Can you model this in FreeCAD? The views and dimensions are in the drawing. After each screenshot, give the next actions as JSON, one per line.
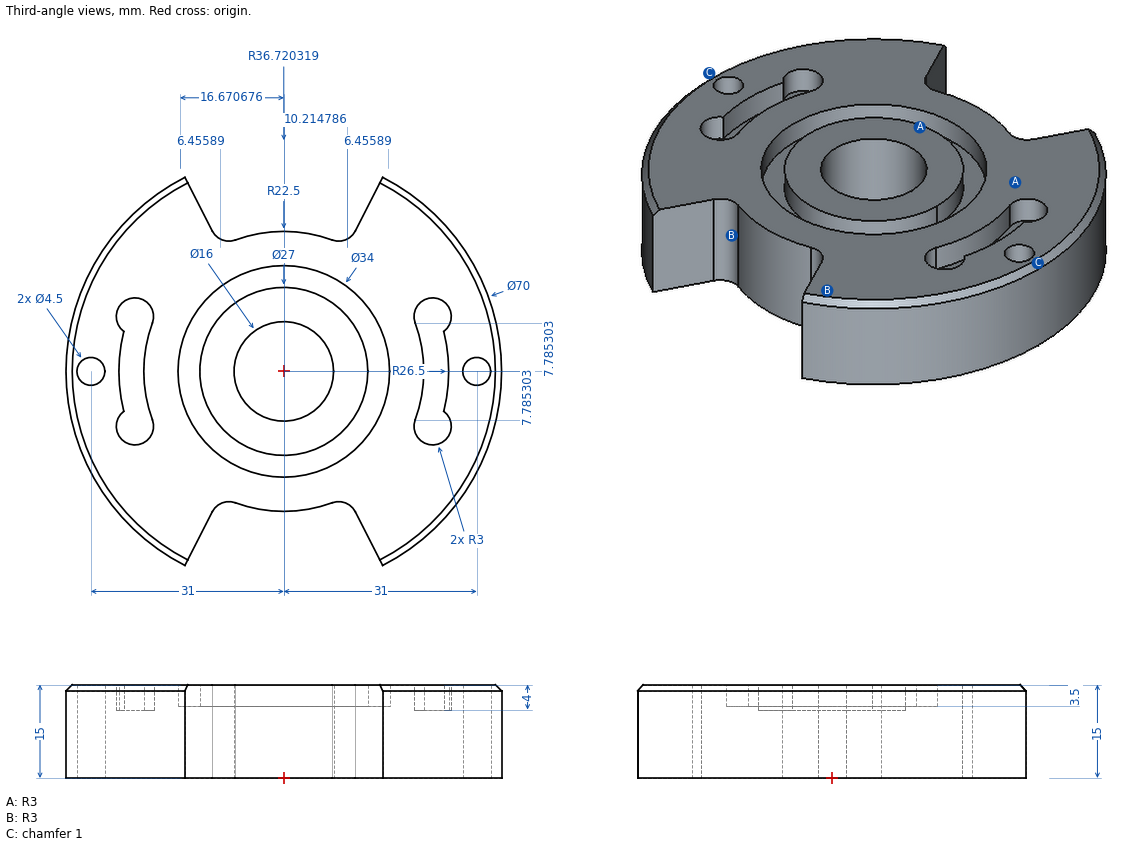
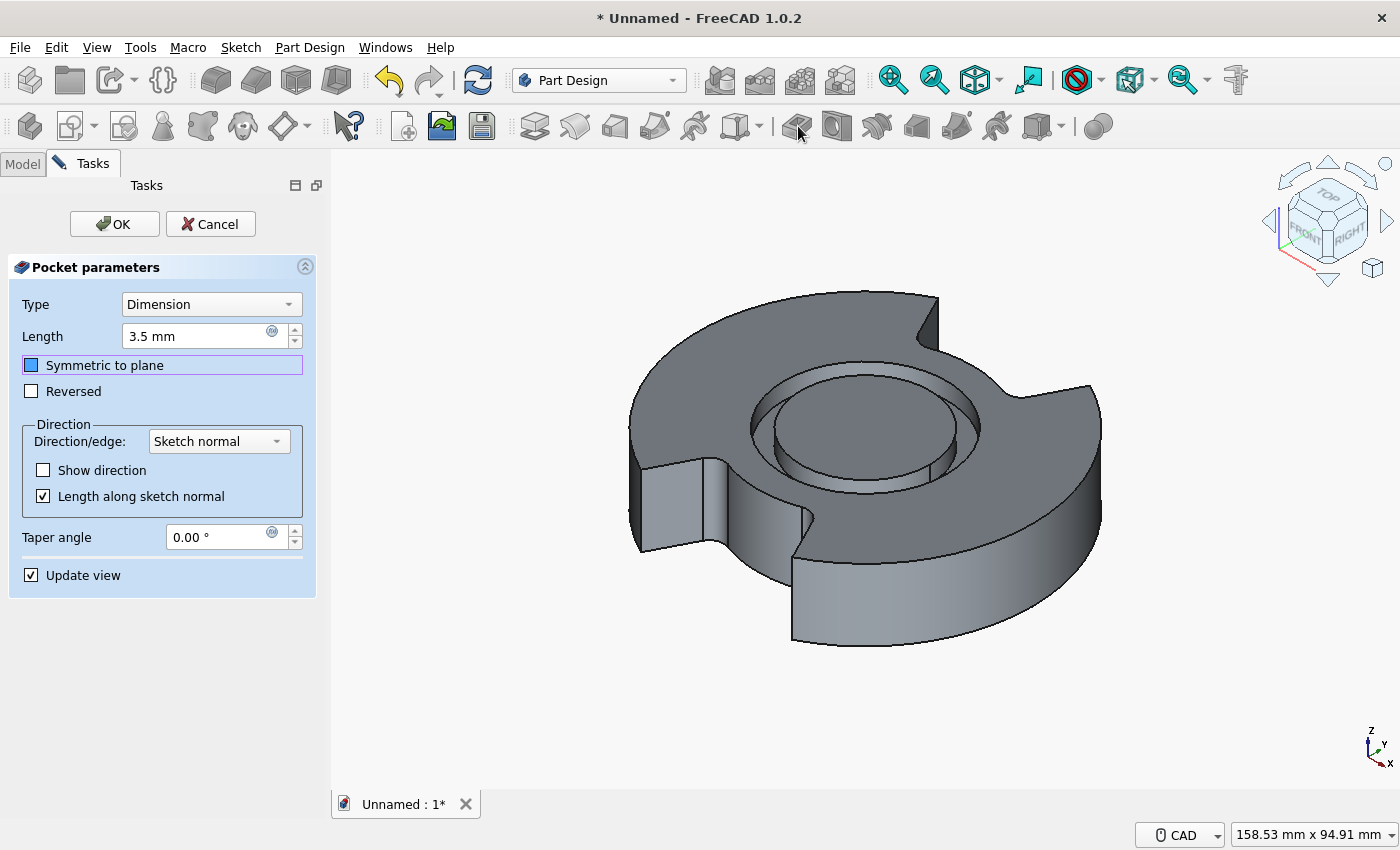
{"action": "left_click", "coordinate": [115, 224]}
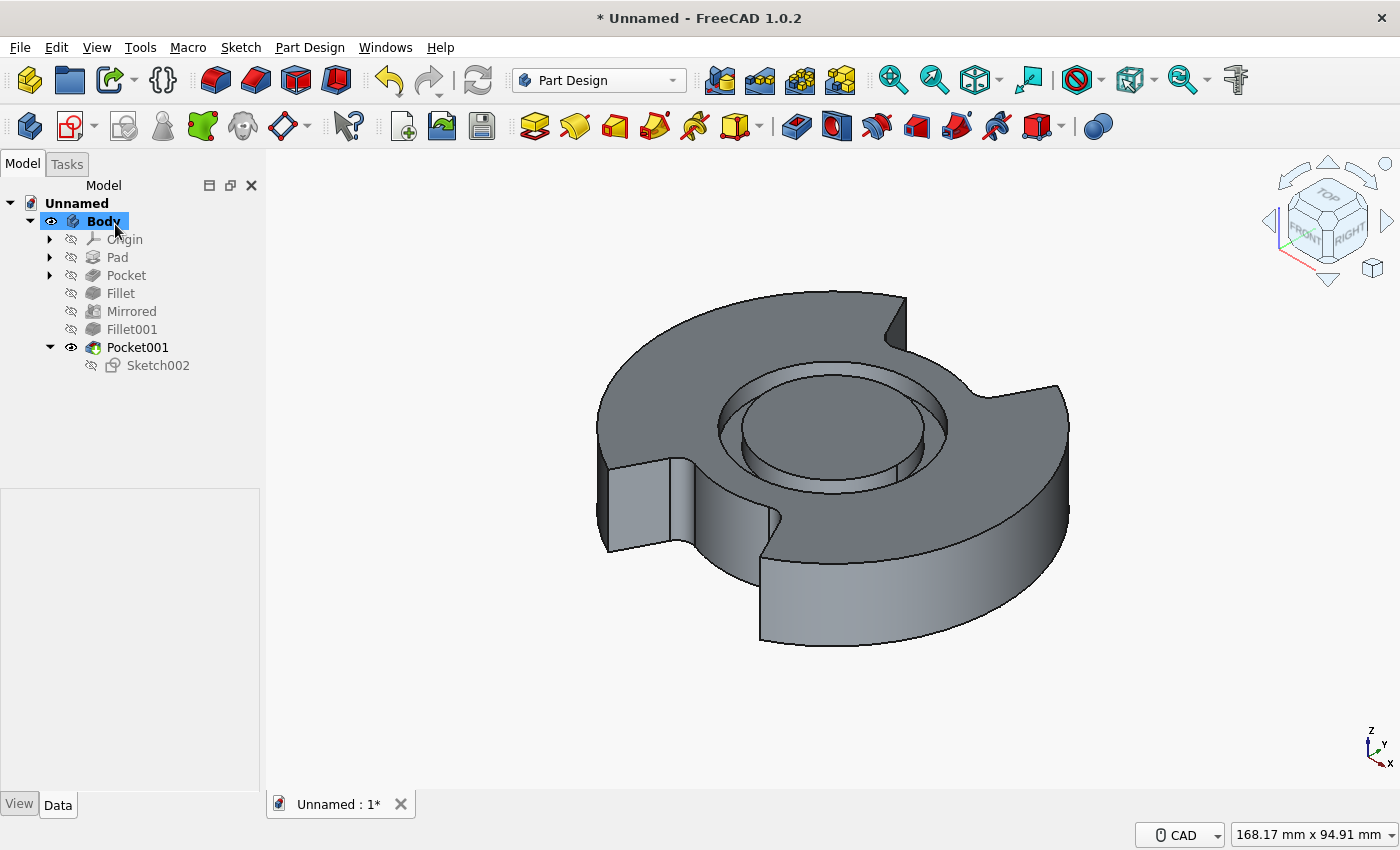
{"action": "left_click", "coordinate": [1013, 433]}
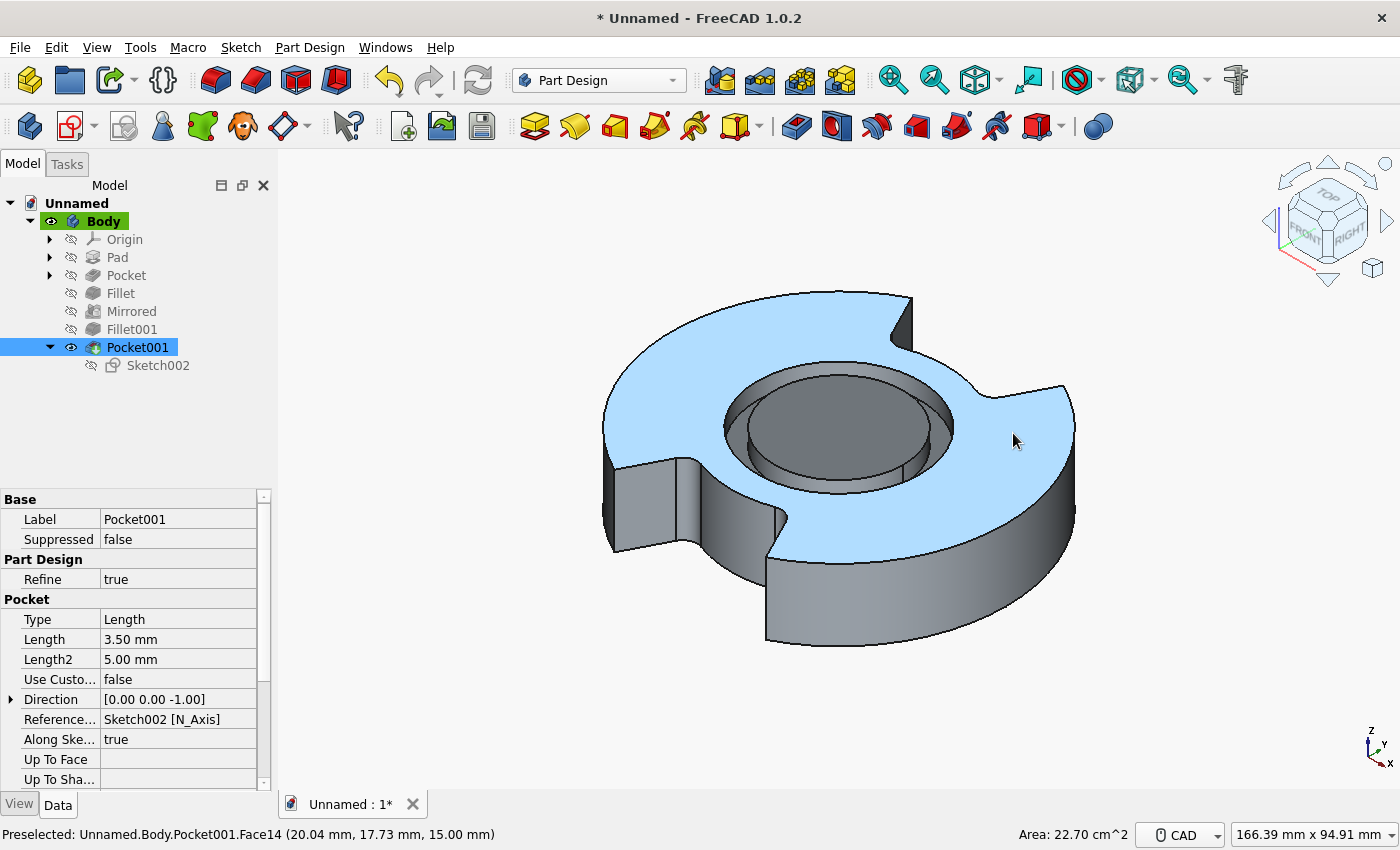
{"action": "left_click", "coordinate": [70, 126]}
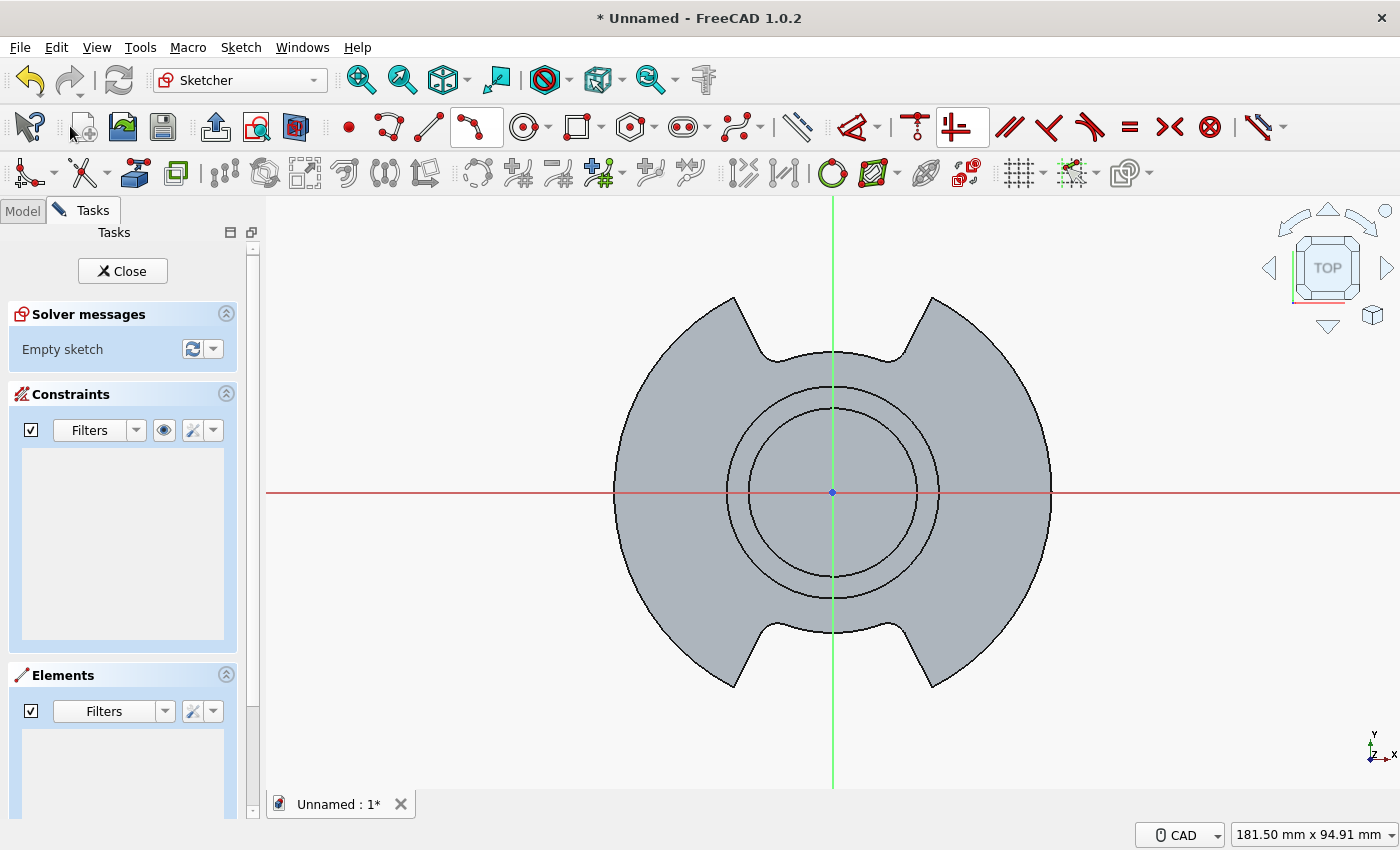
{"action": "scroll", "coordinate": [1004, 493], "scroll_direction": "up", "scroll_amount": 5}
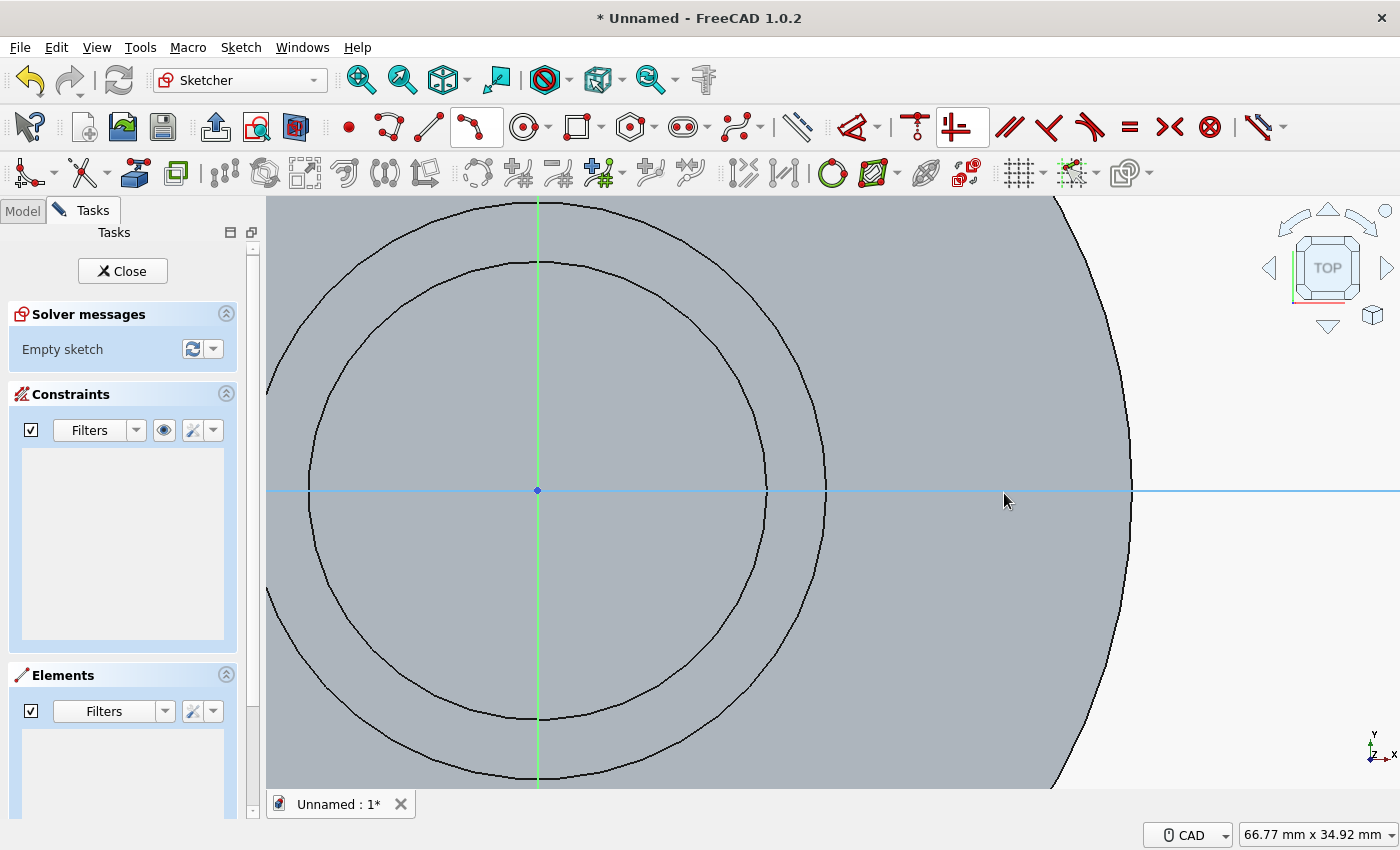
{"action": "left_click", "coordinate": [470, 128]}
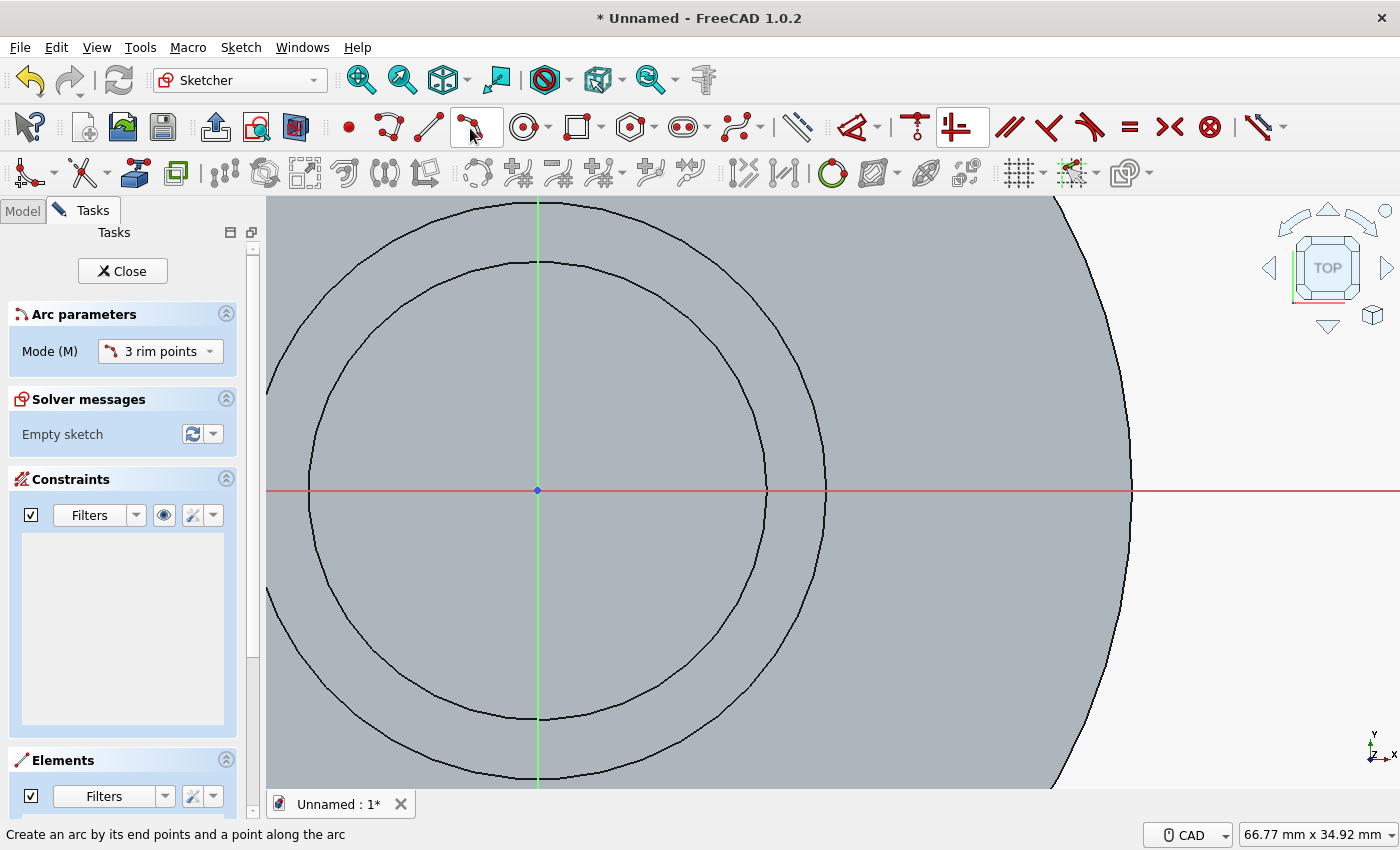
{"action": "left_click", "coordinate": [896, 359]}
{"action": "left_click", "coordinate": [896, 623]}
{"action": "left_click", "coordinate": [919, 518]}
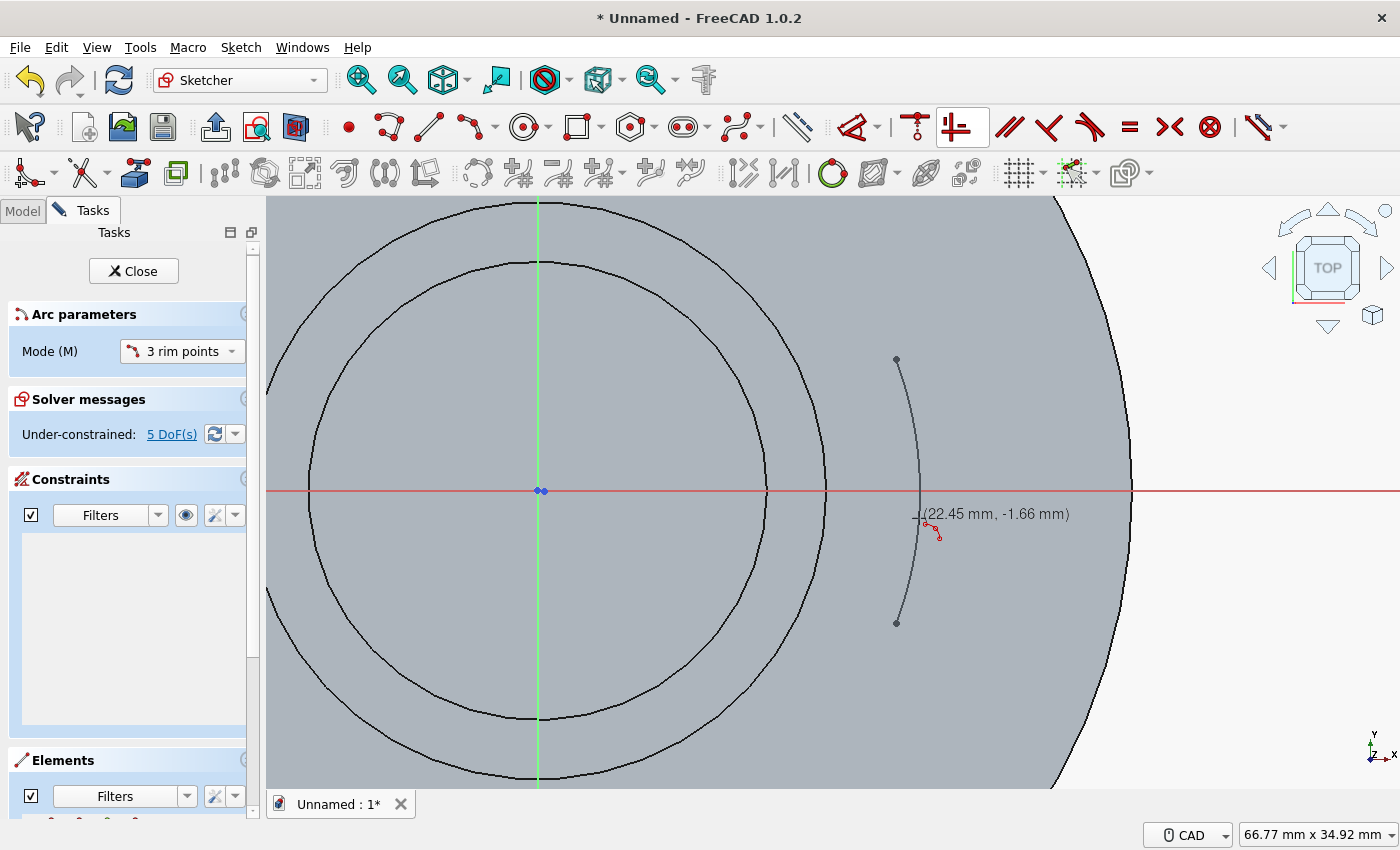
{"action": "left_click", "coordinate": [896, 624]}
{"action": "left_click", "coordinate": [974, 600]}
{"action": "left_click", "coordinate": [959, 689]}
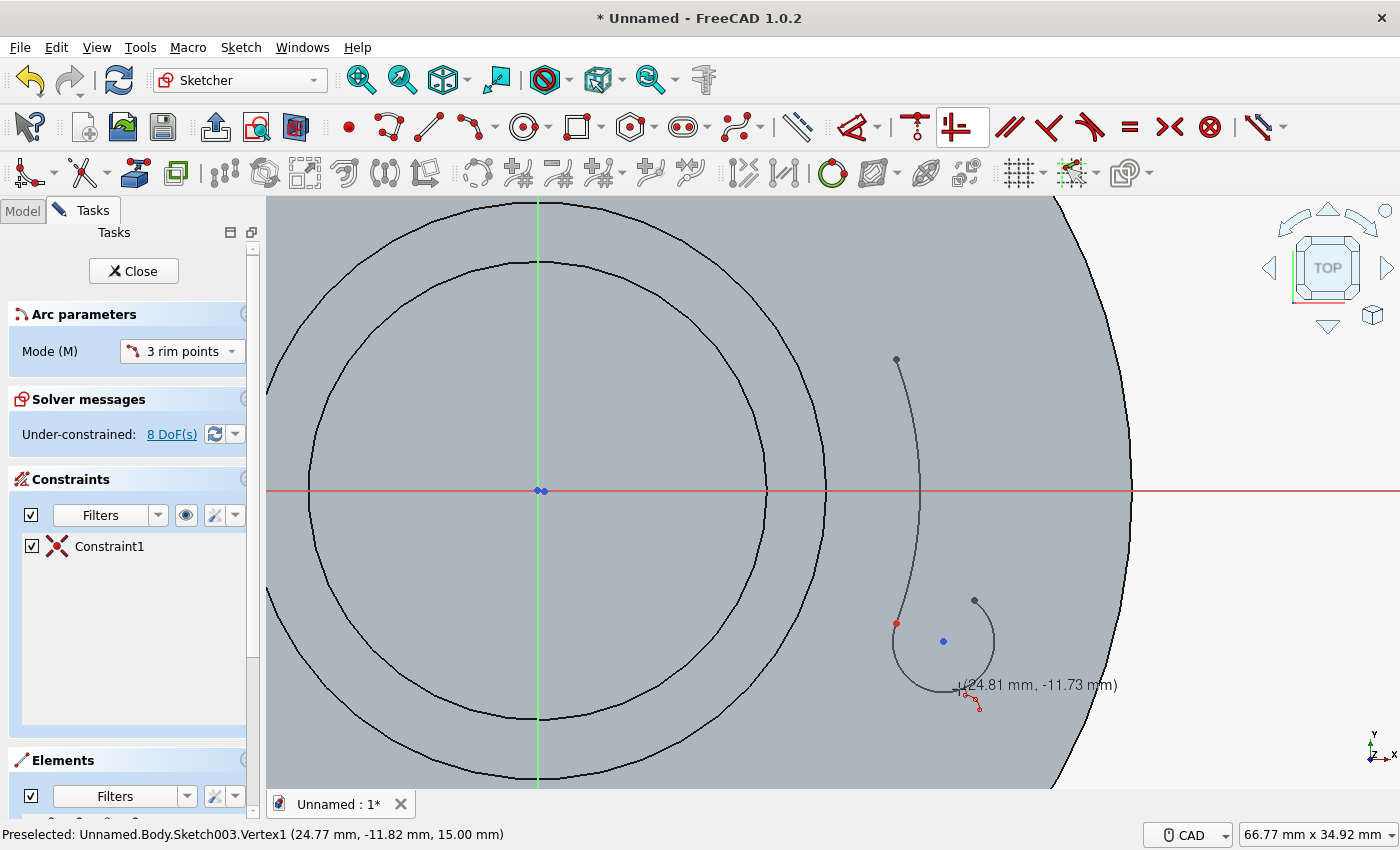
{"action": "left_click", "coordinate": [974, 601]}
{"action": "left_click", "coordinate": [974, 382]}